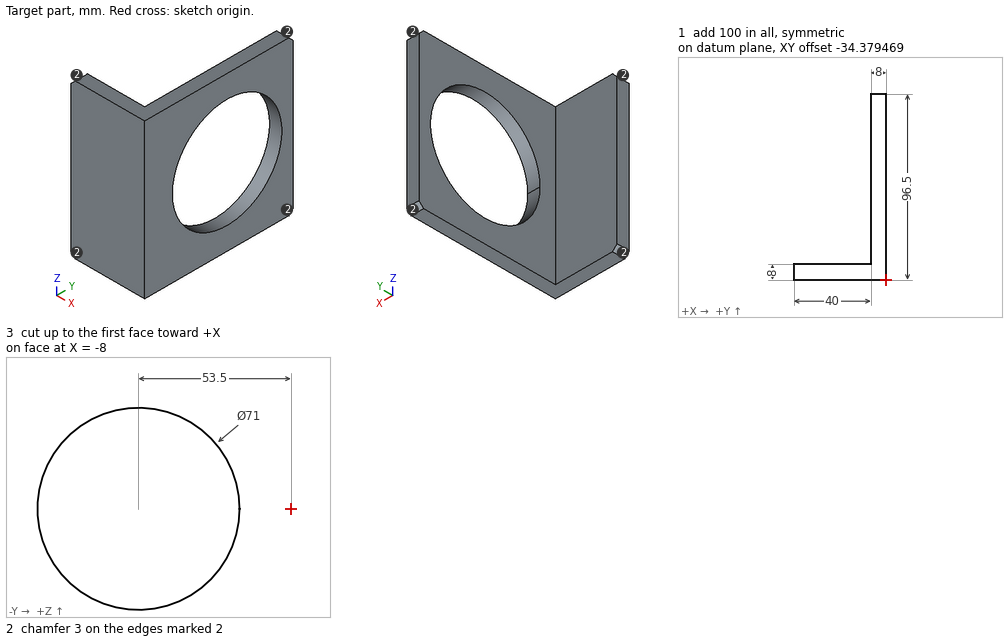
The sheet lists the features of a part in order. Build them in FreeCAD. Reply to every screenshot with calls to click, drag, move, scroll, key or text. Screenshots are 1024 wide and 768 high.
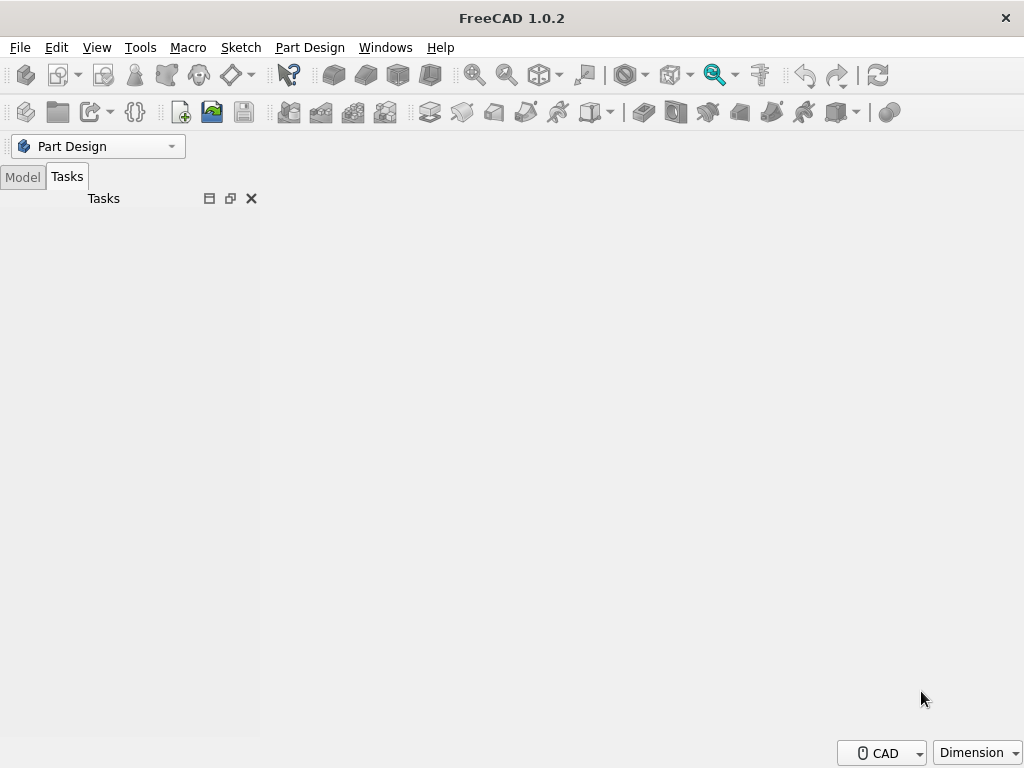
click(180, 112)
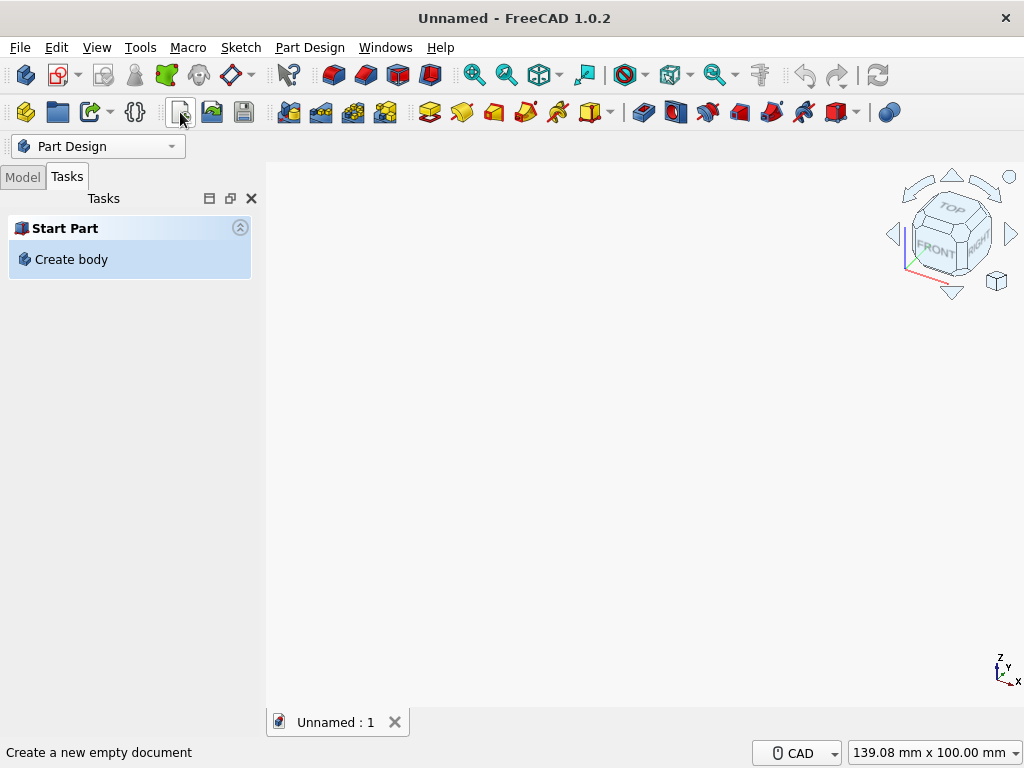
click(26, 76)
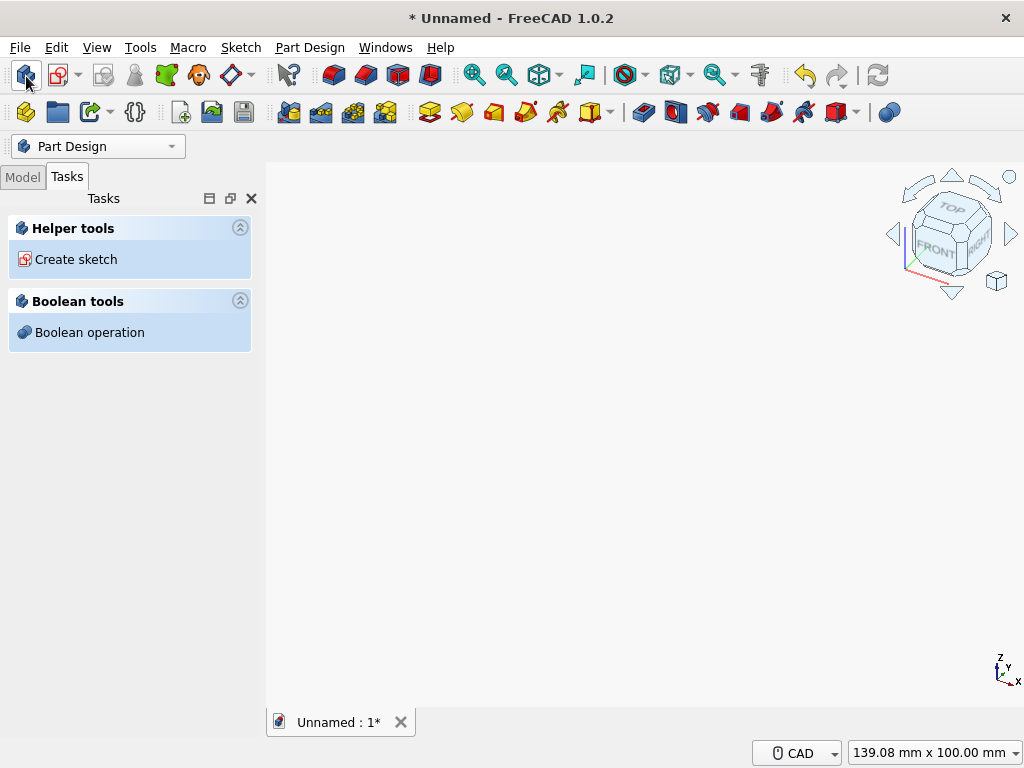
click(23, 176)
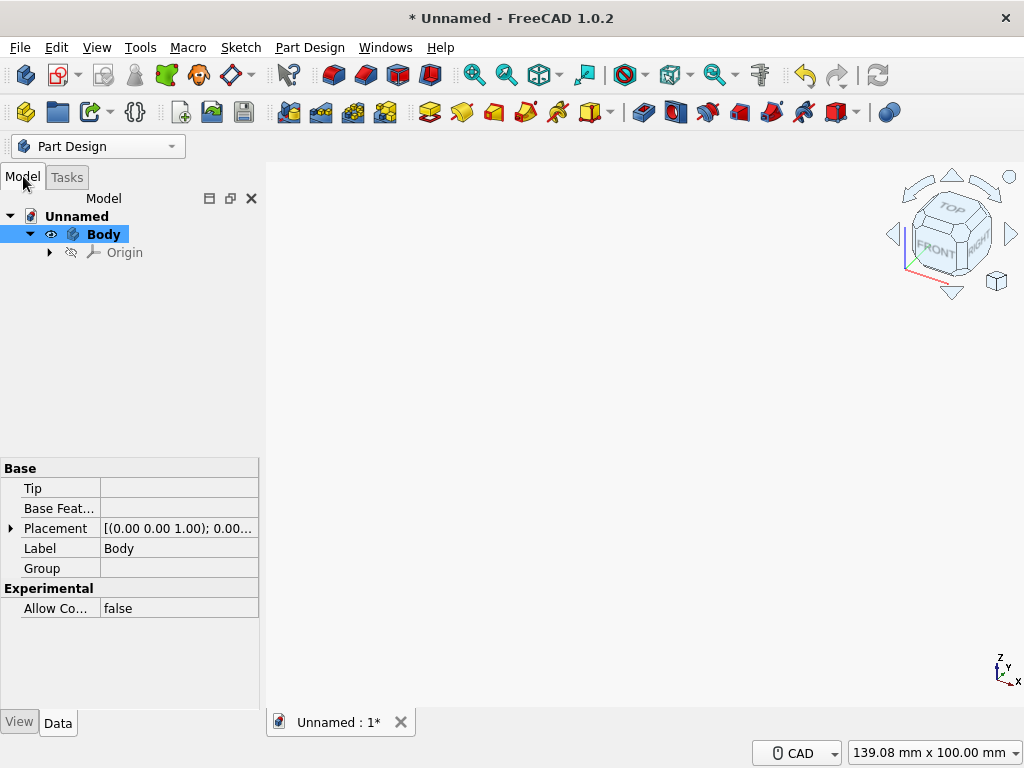
click(50, 252)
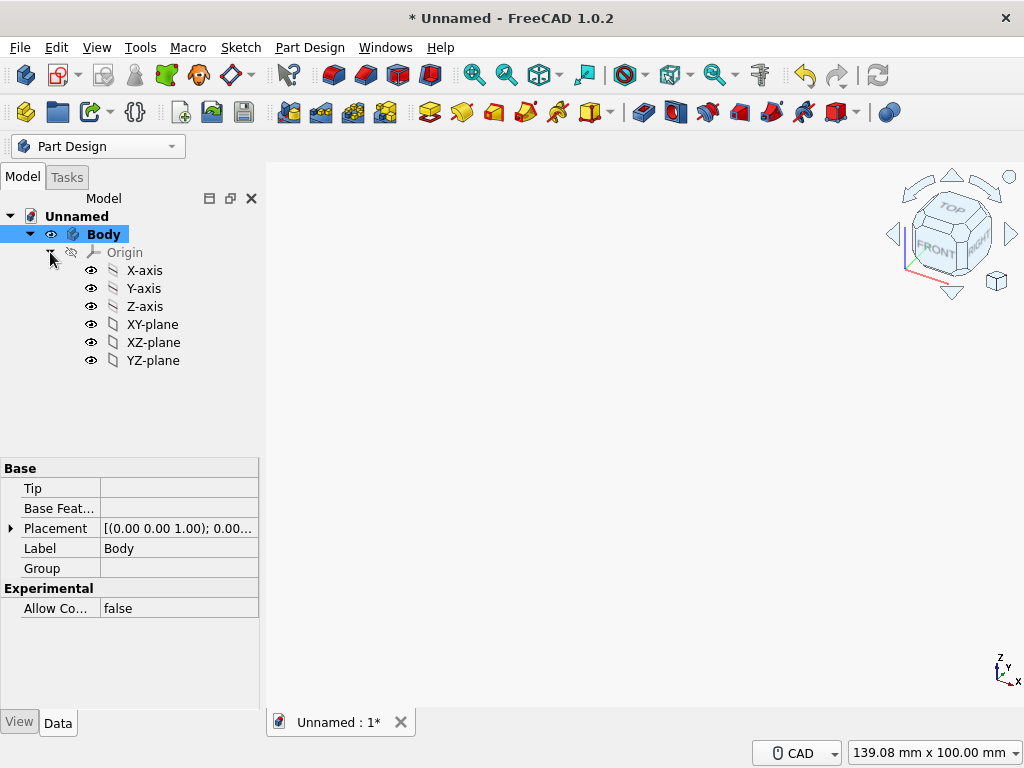
click(136, 324)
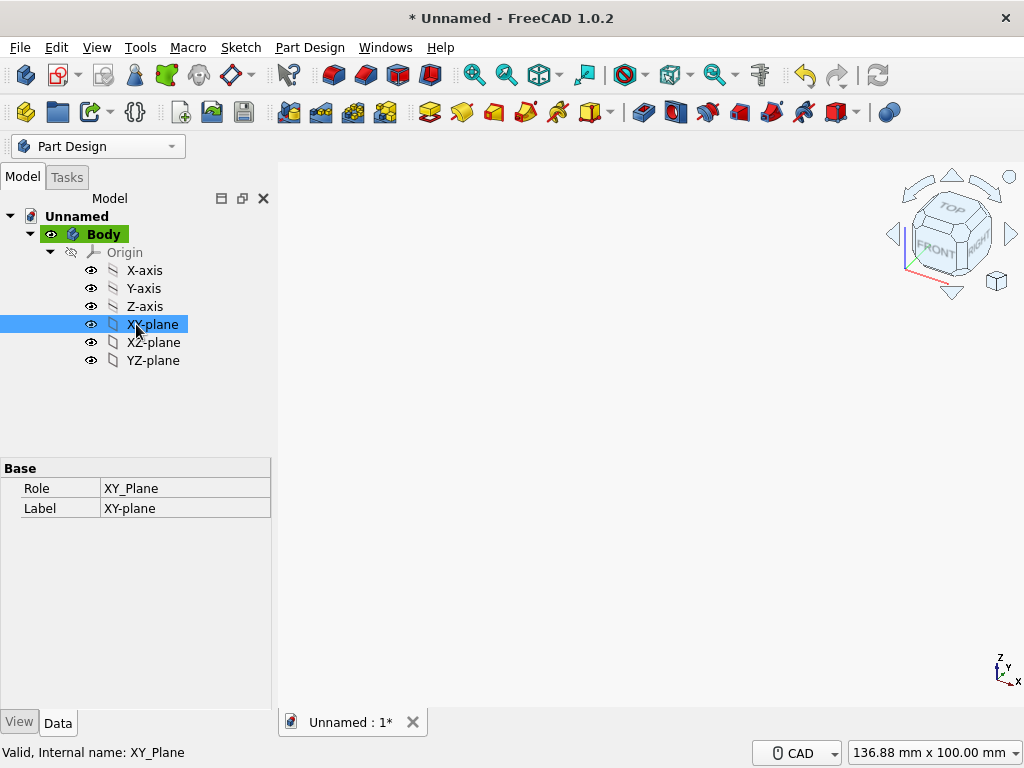
click(232, 76)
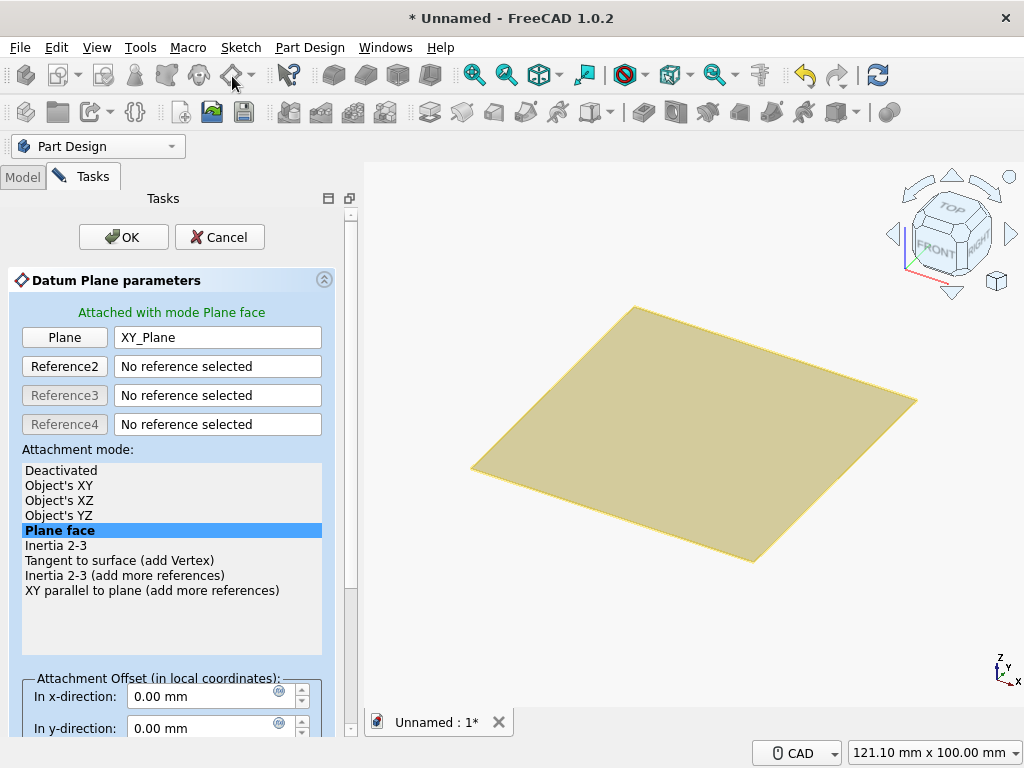
scroll(351, 472, down, 2)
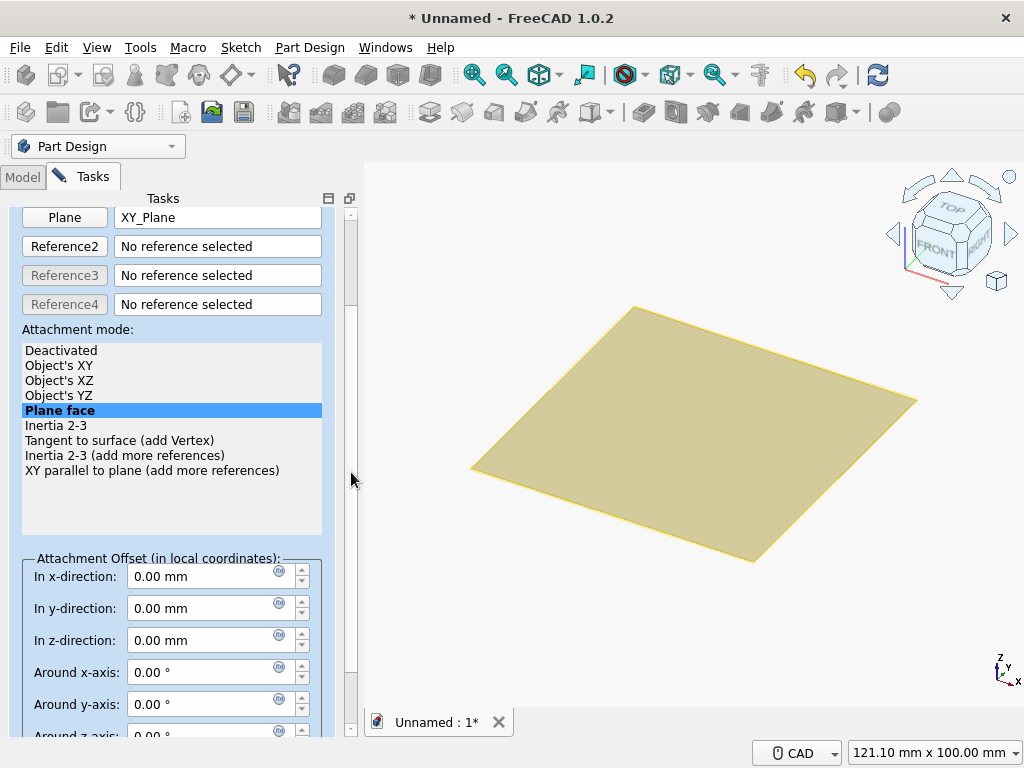
triple_click(210, 640)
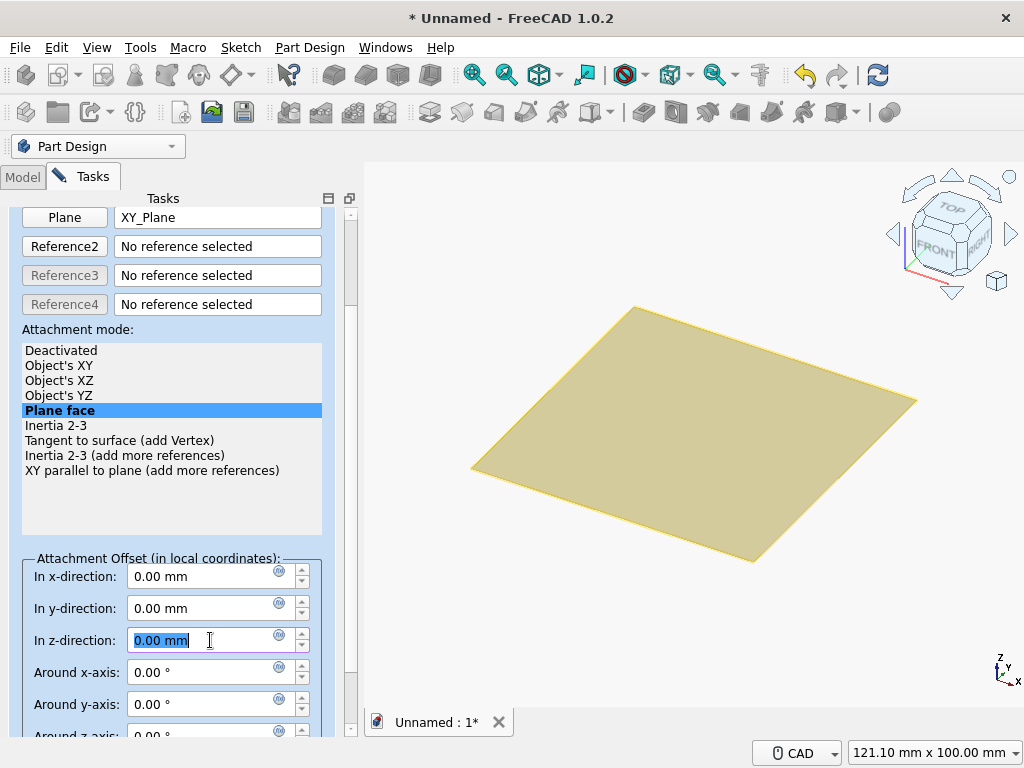
text(-34.379469)
key(Tab)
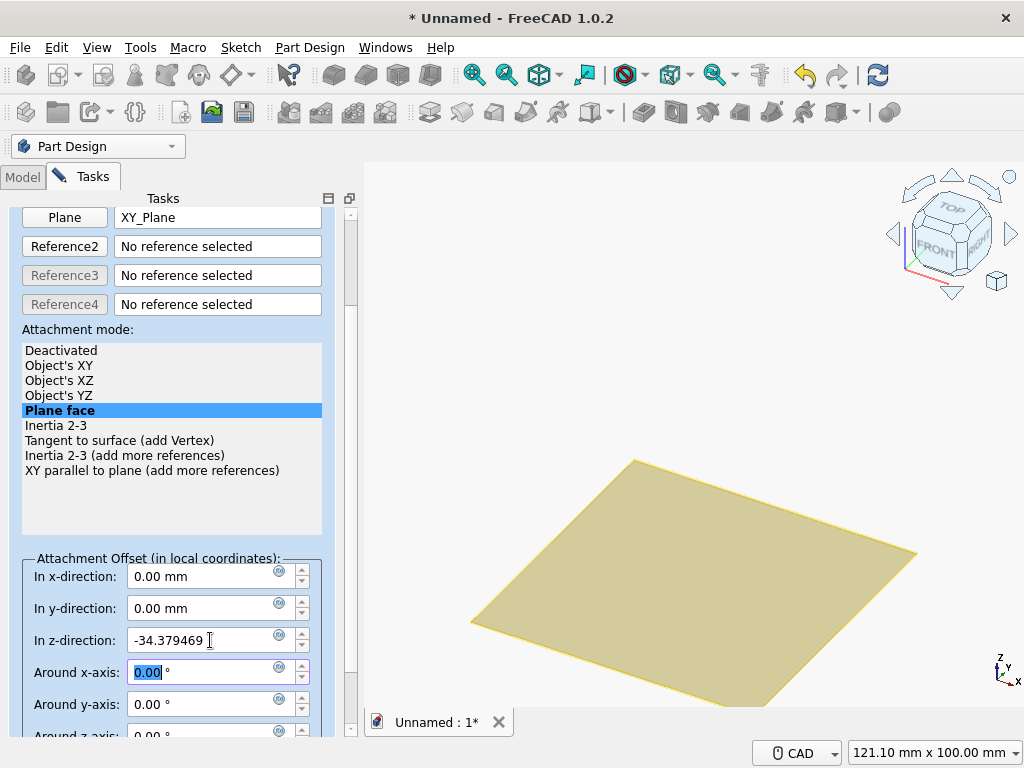
scroll(351, 472, up, 3)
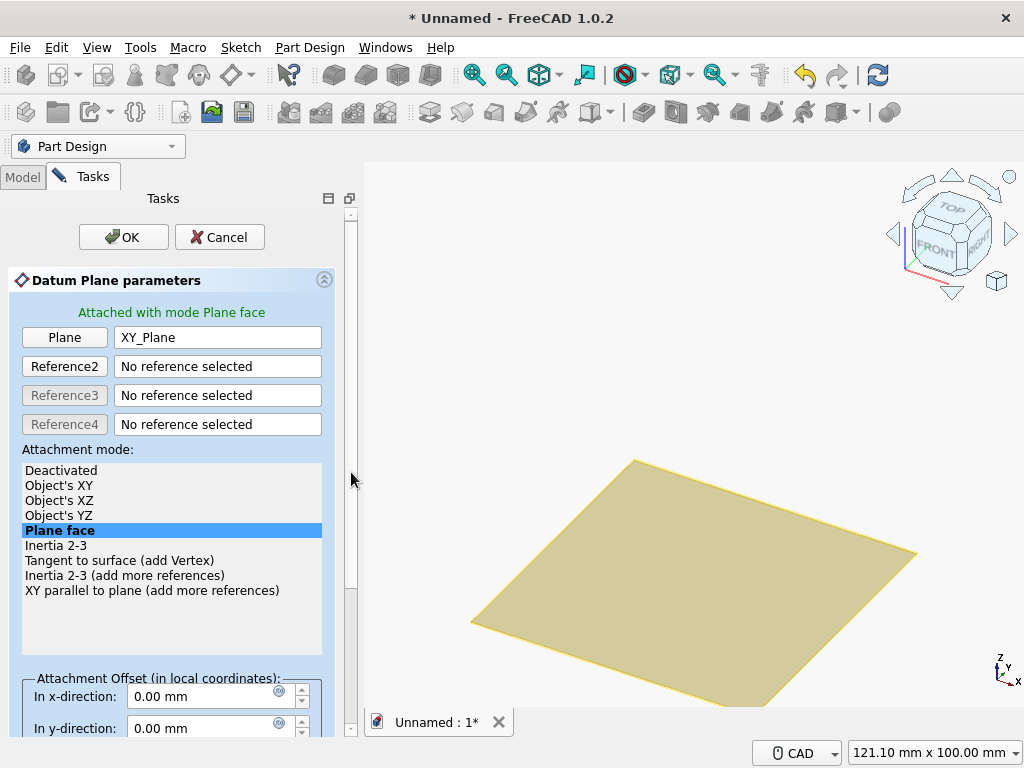
click(124, 237)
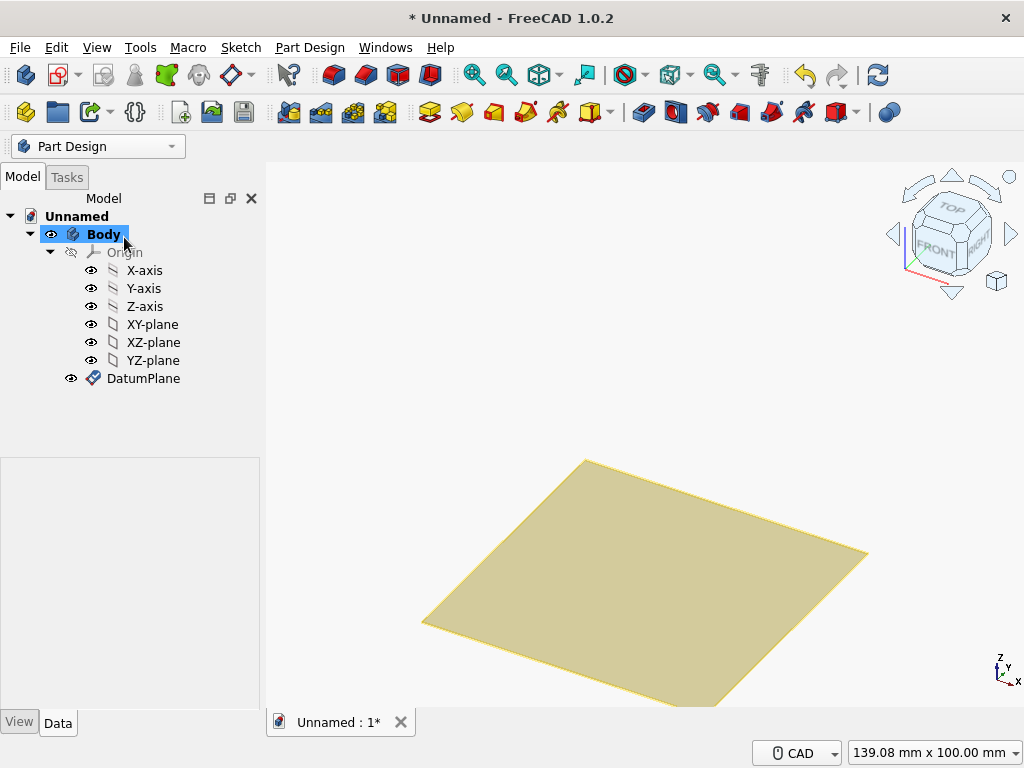
click(116, 378)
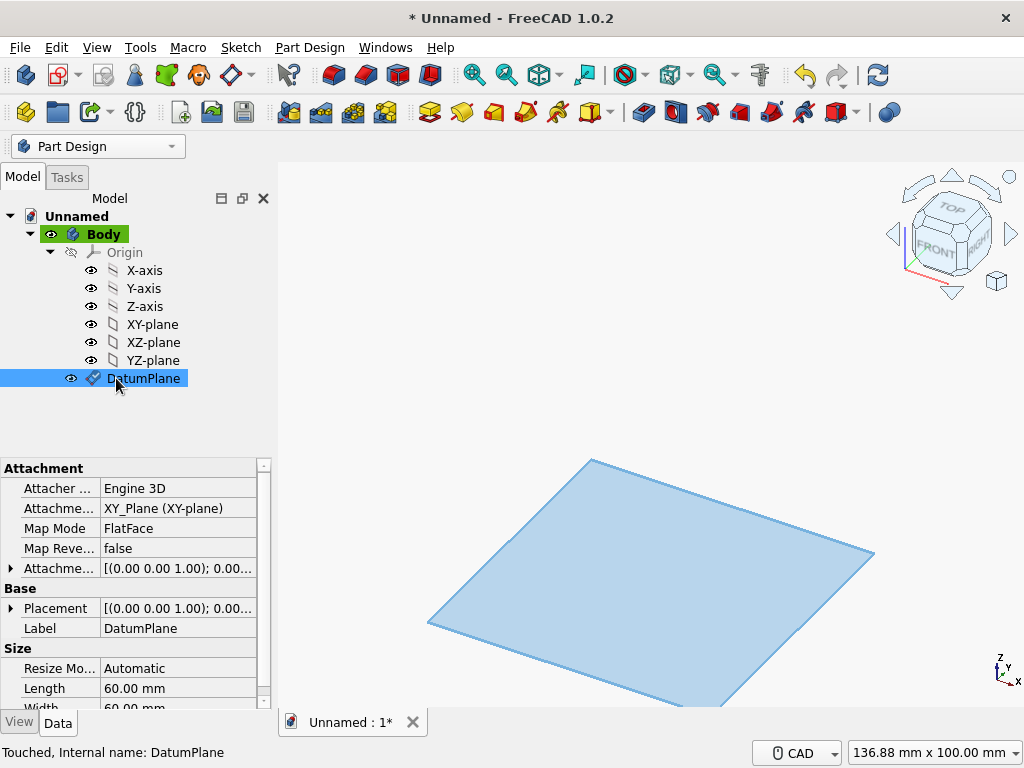
click(58, 76)